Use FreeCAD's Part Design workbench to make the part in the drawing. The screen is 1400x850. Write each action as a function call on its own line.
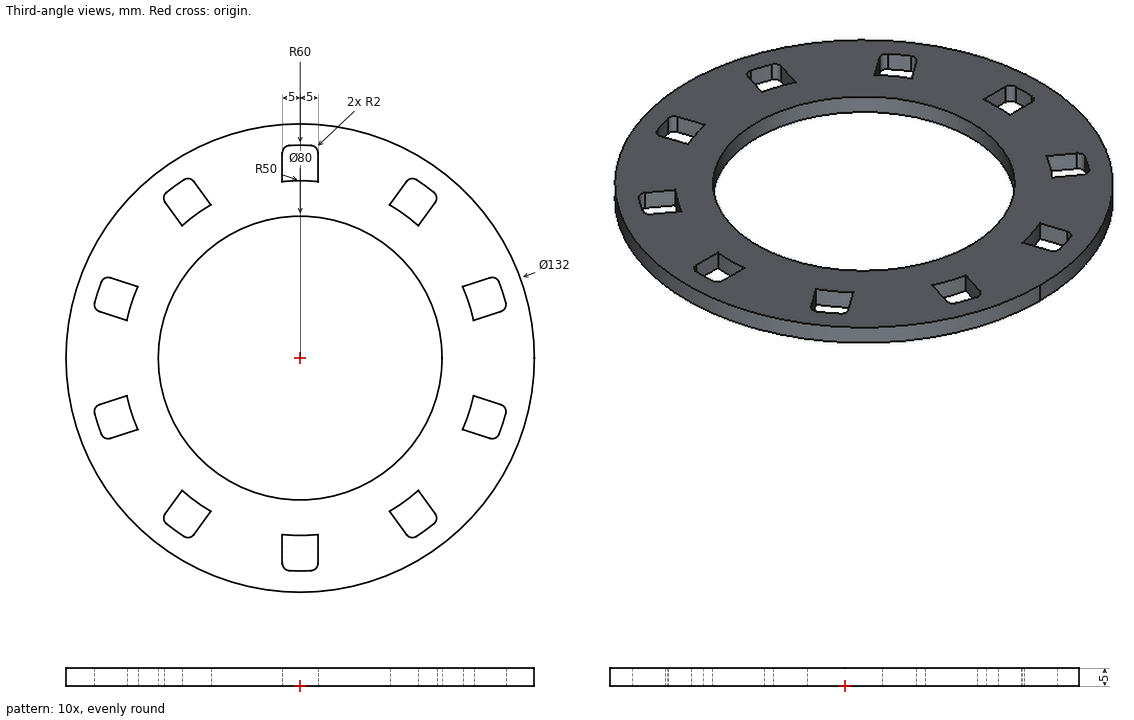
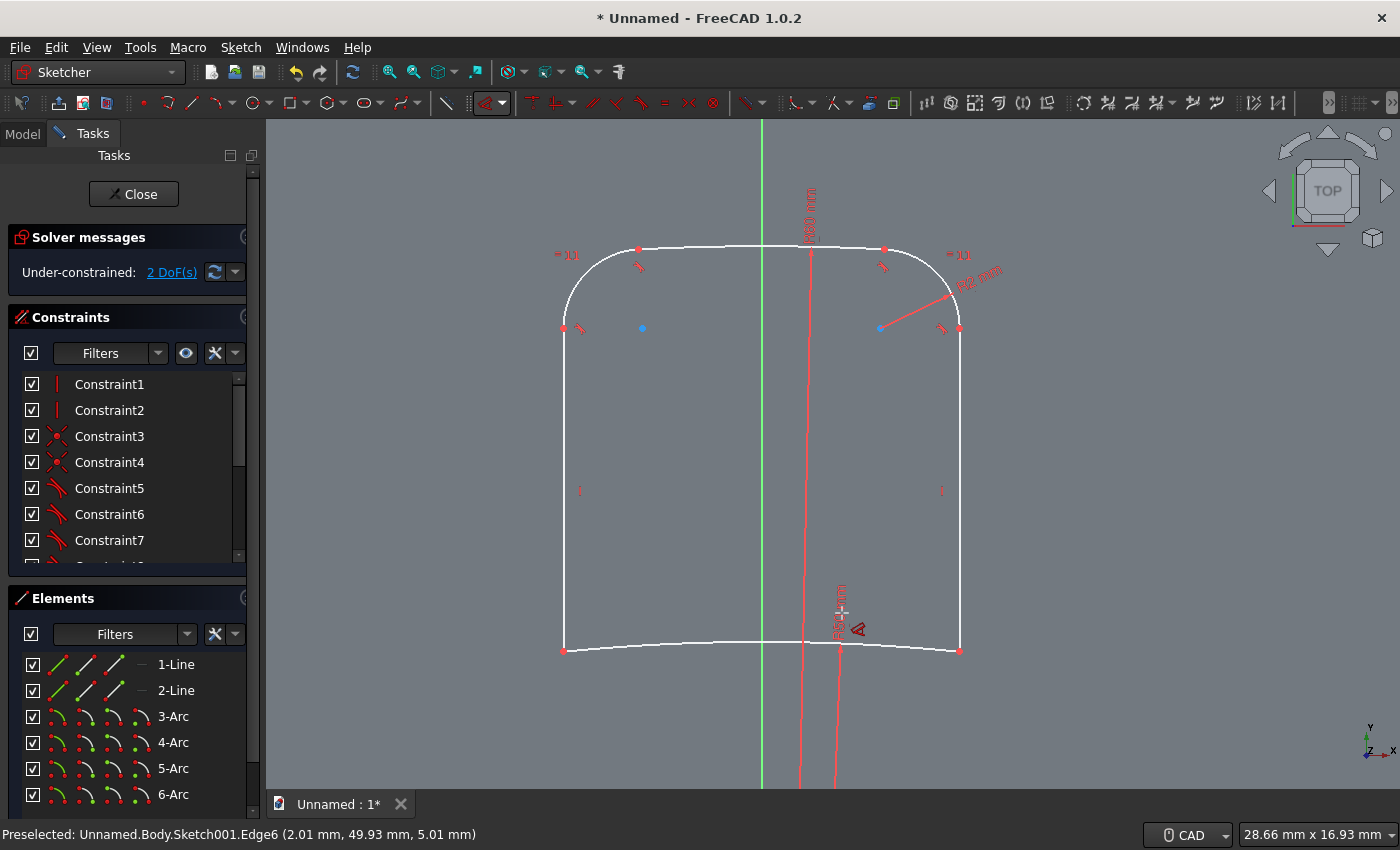
click(960, 652)
click(930, 618)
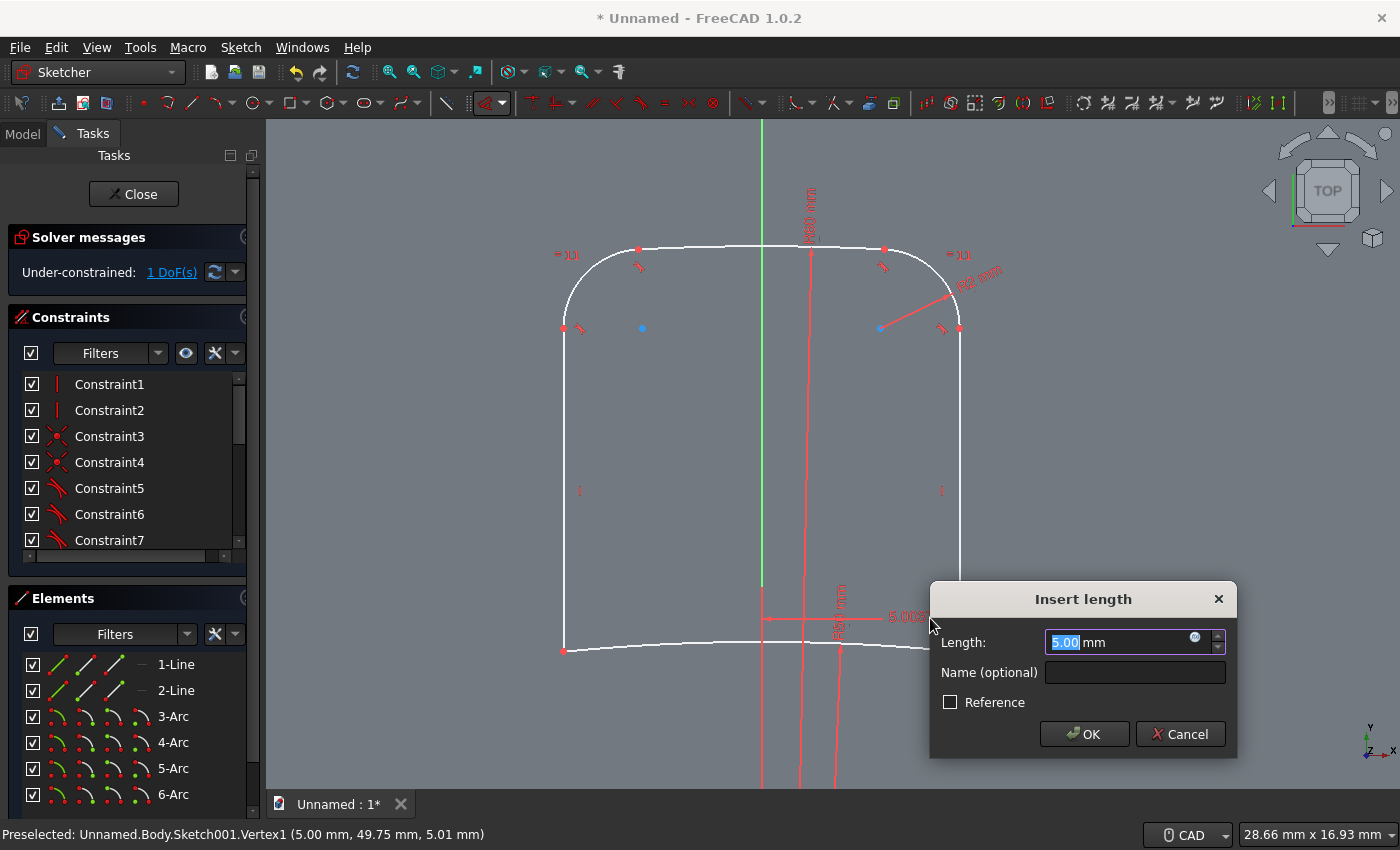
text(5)
key(Return)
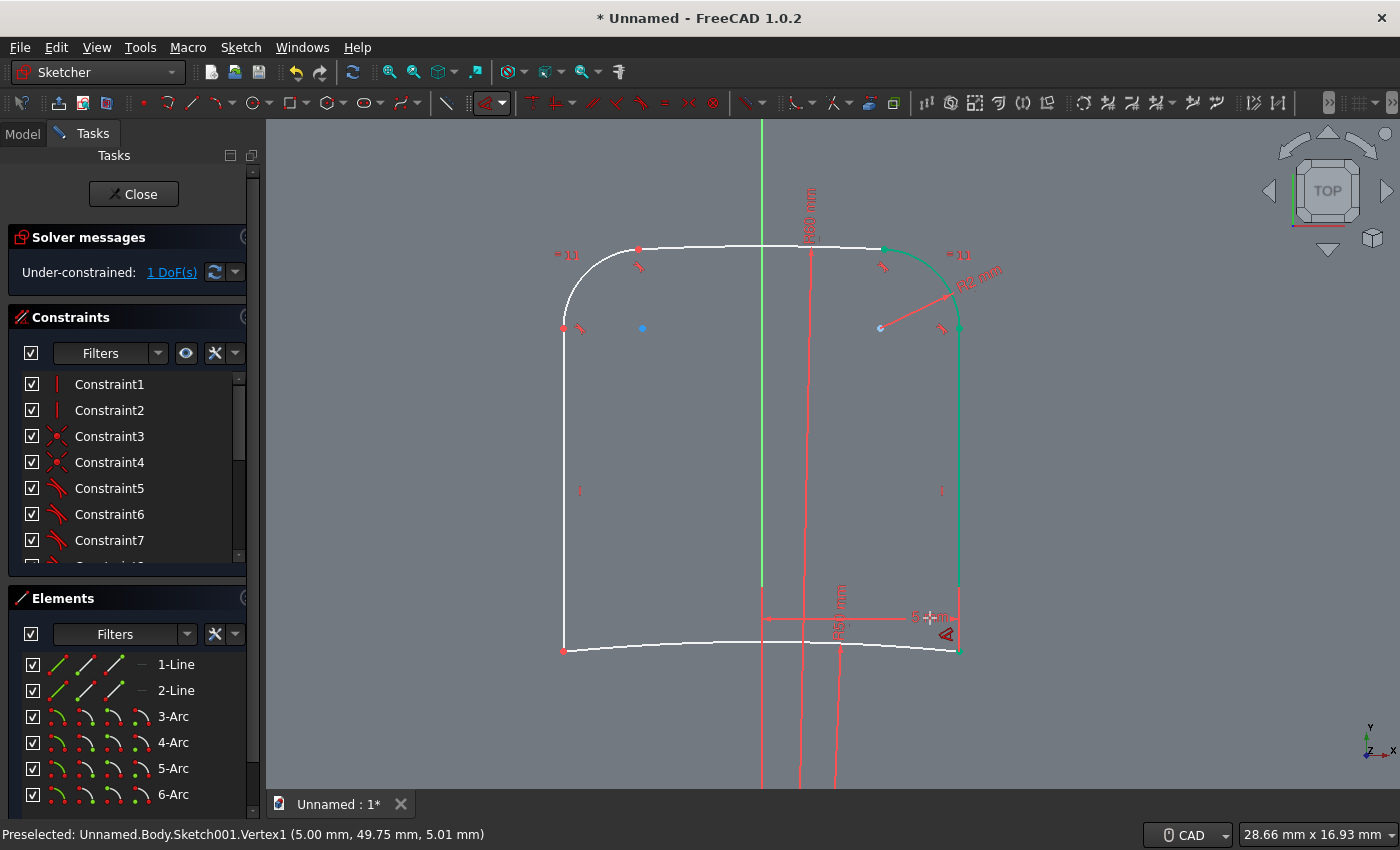
click(564, 328)
click(663, 294)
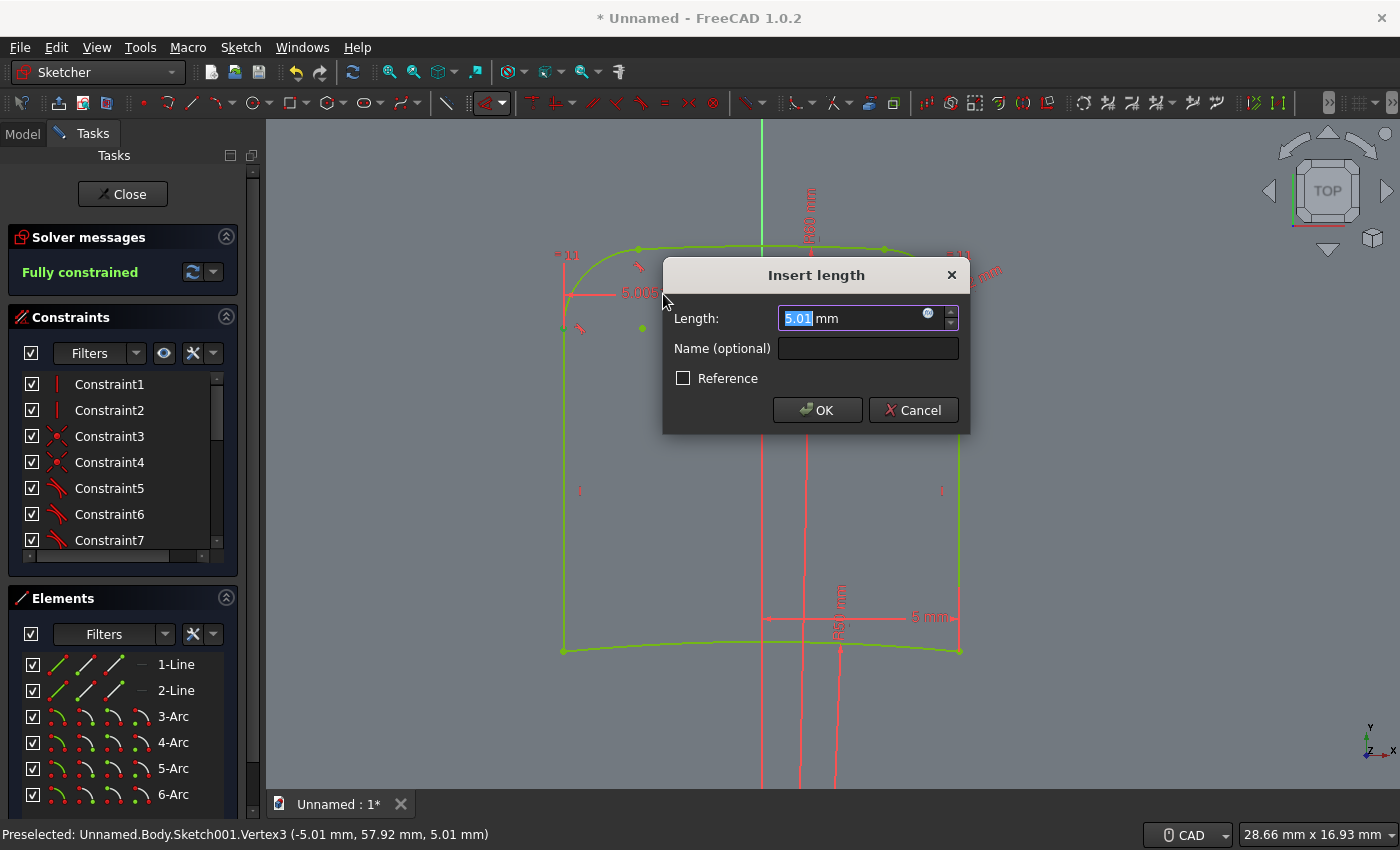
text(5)
key(Return)
key(Escape)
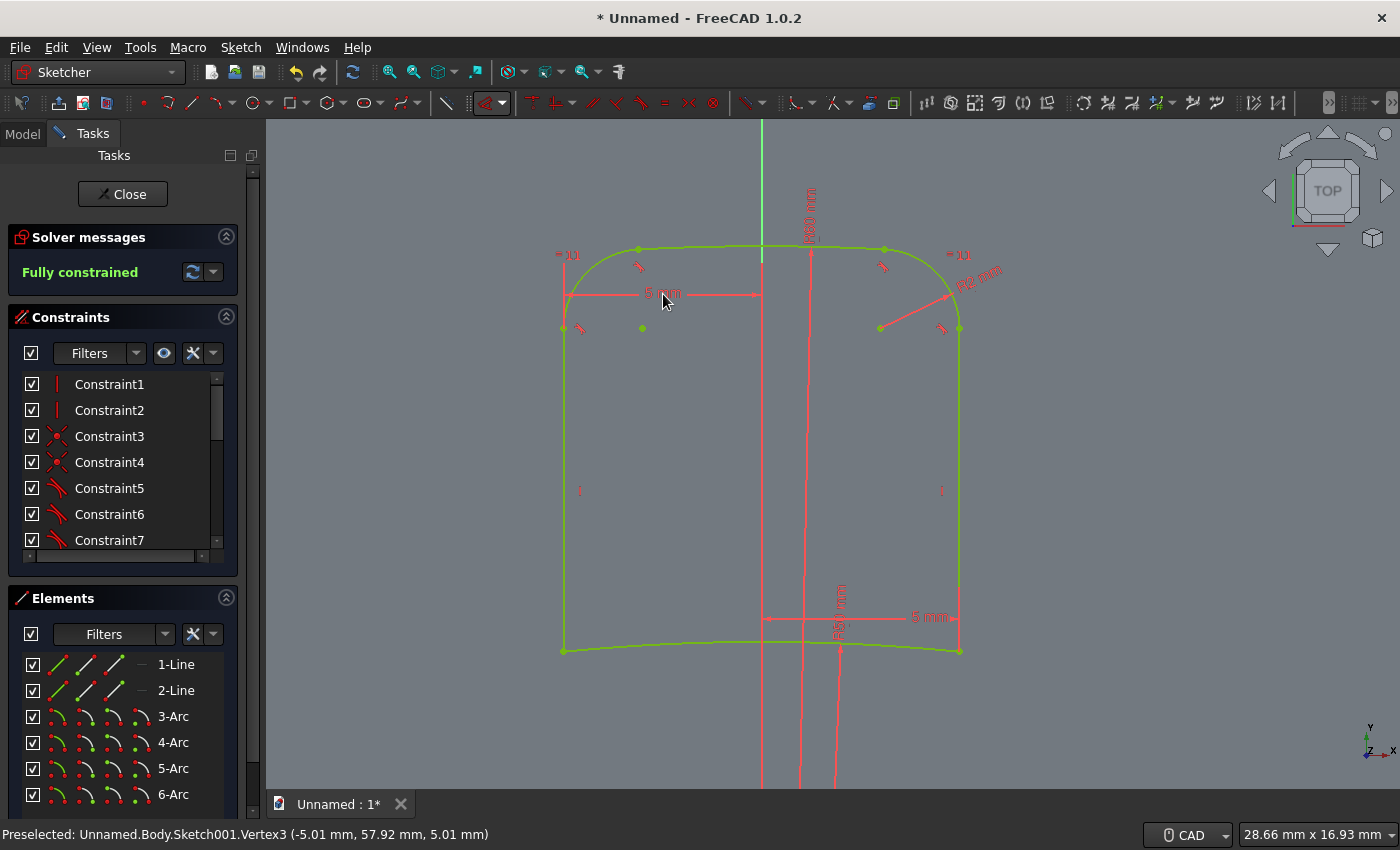
click(123, 194)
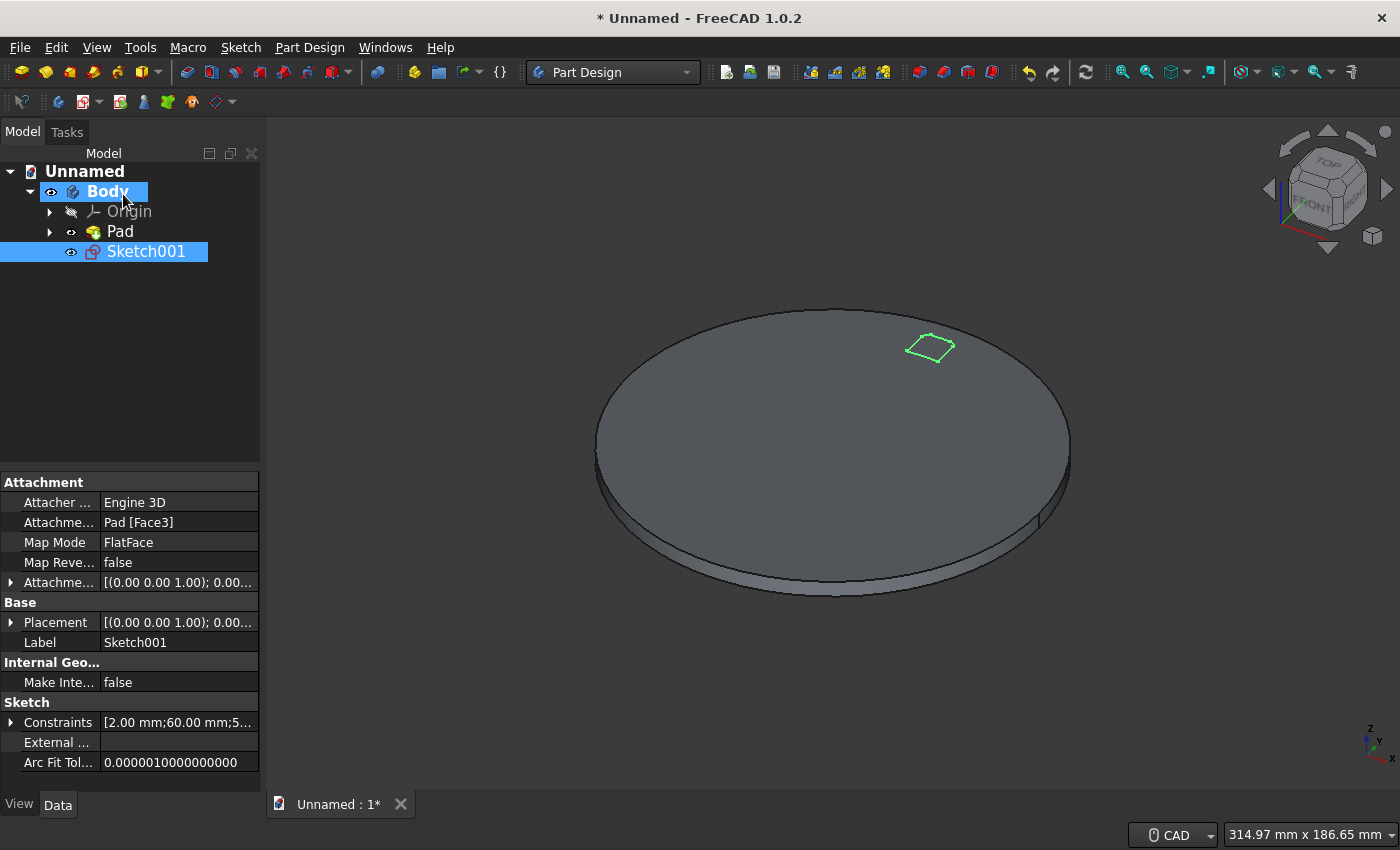
click(188, 72)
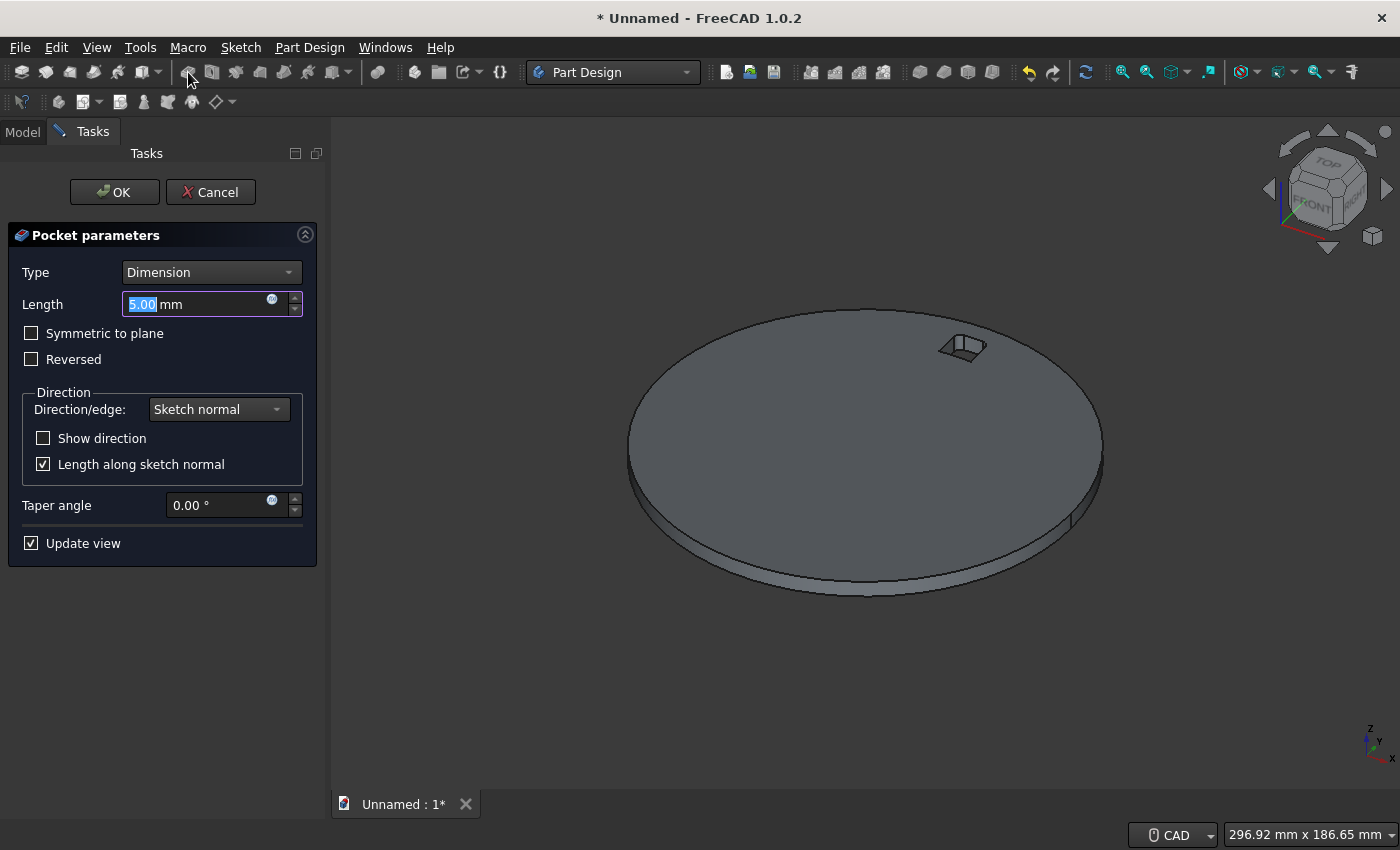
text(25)
key(Tab)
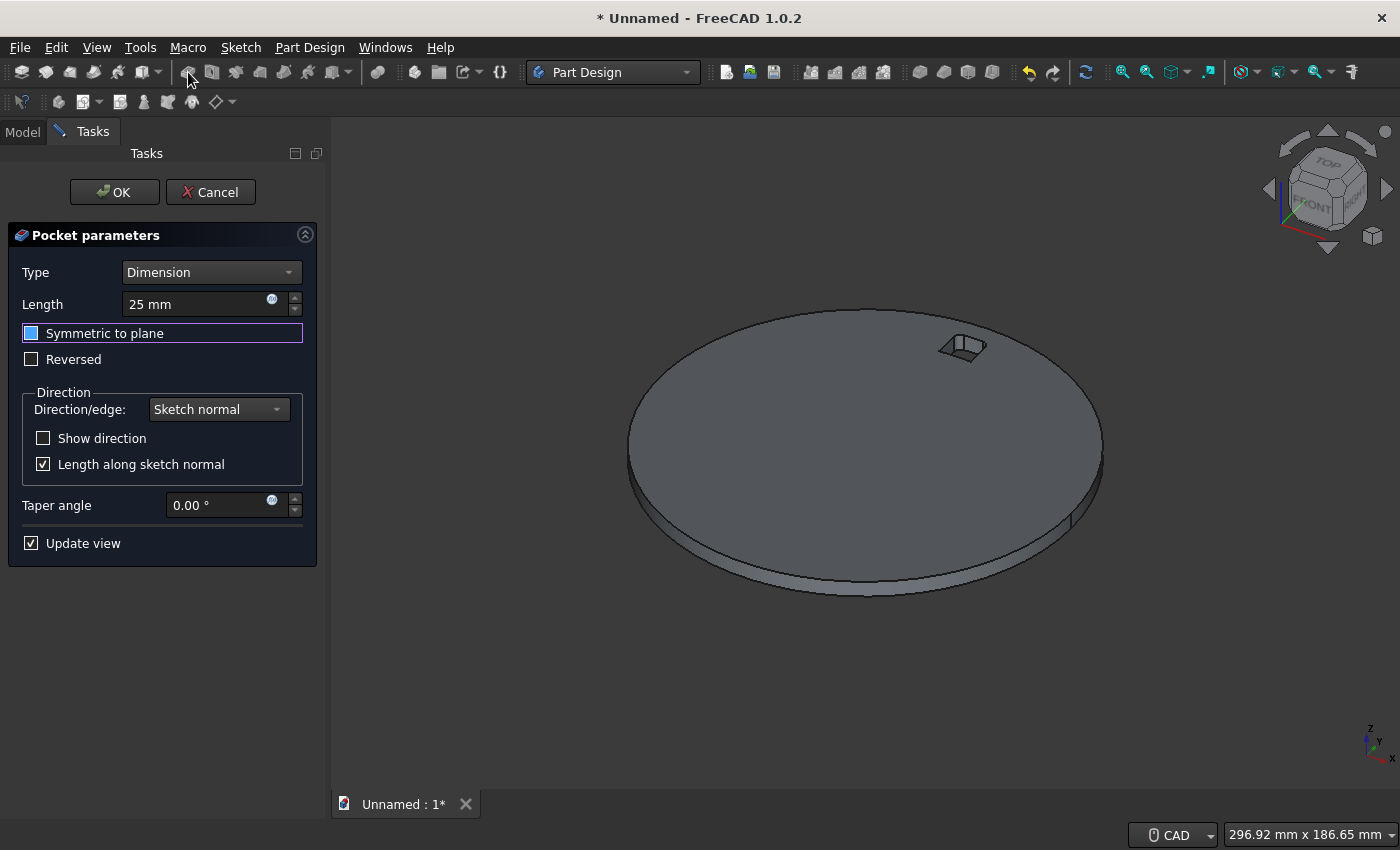
click(115, 192)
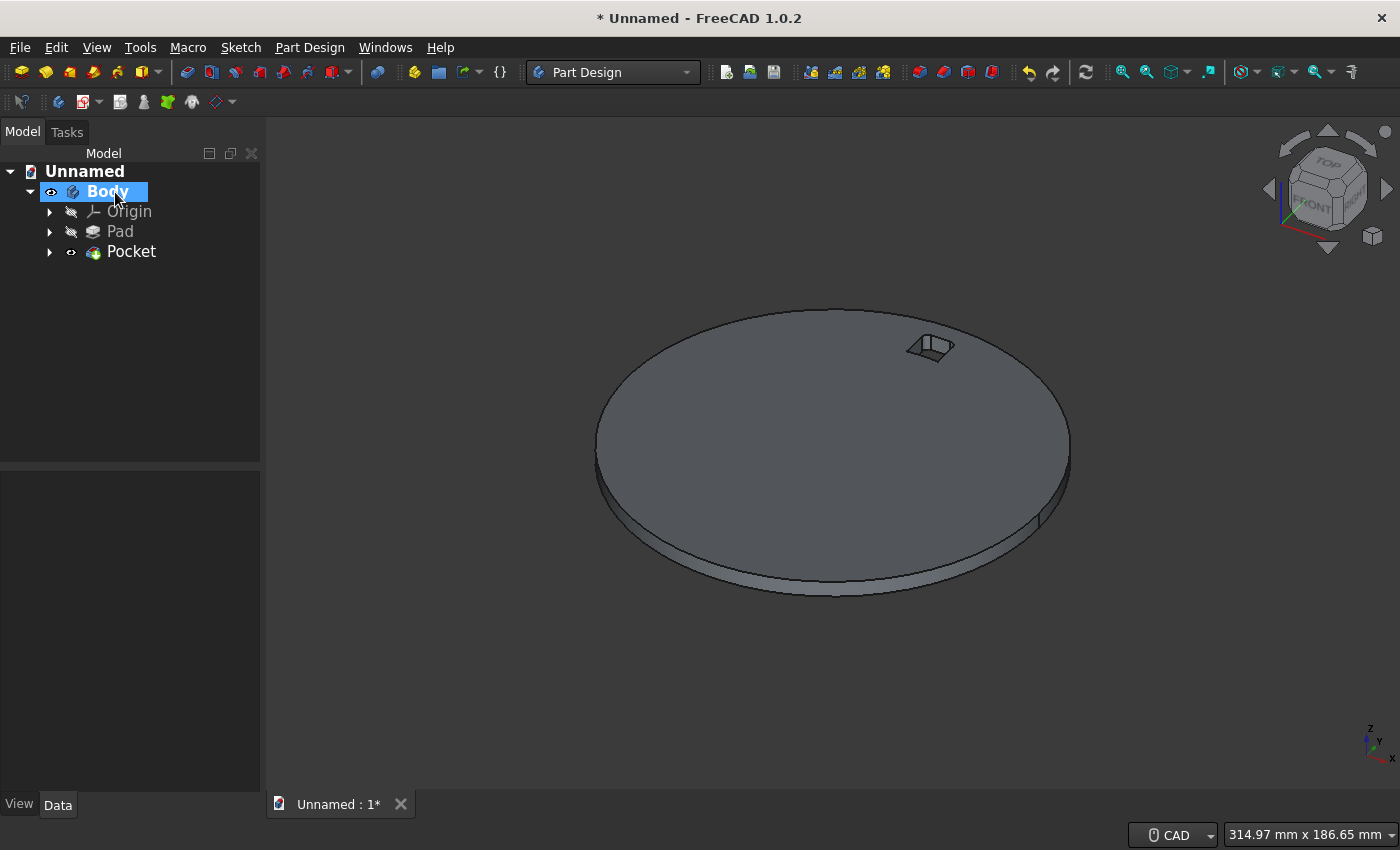
click(116, 252)